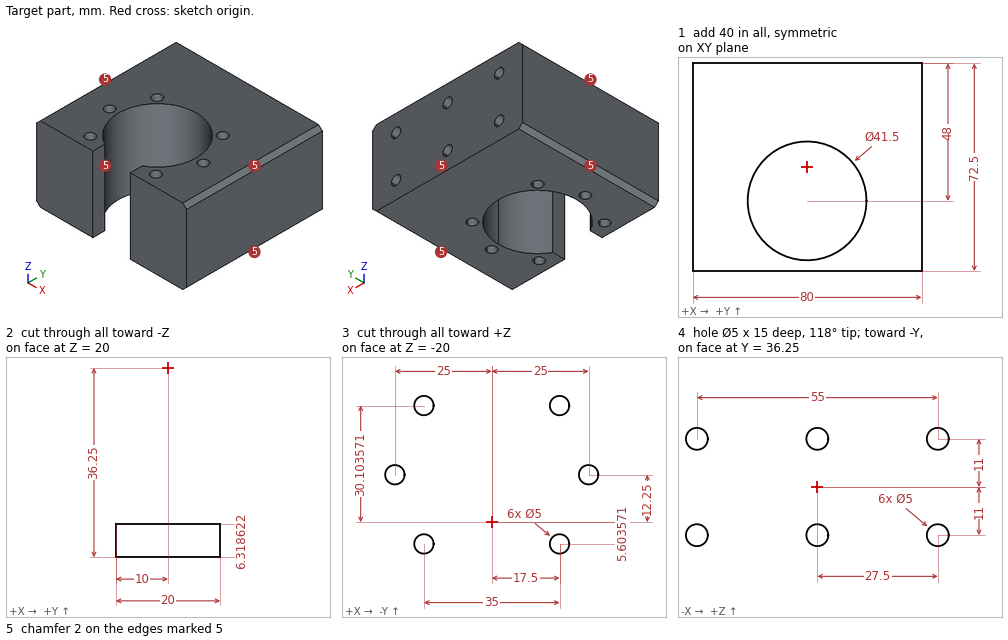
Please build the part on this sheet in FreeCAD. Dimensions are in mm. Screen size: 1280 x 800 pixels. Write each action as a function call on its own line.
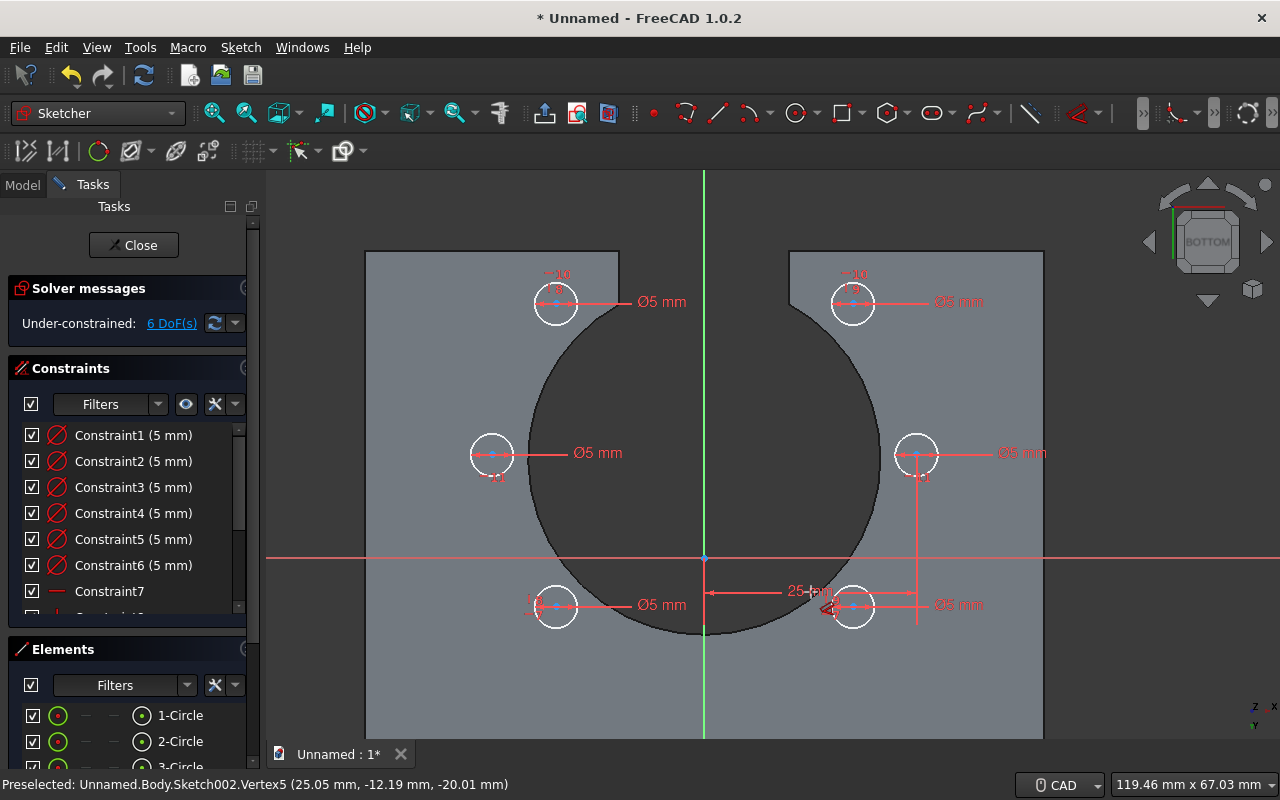
click(492, 455)
click(598, 592)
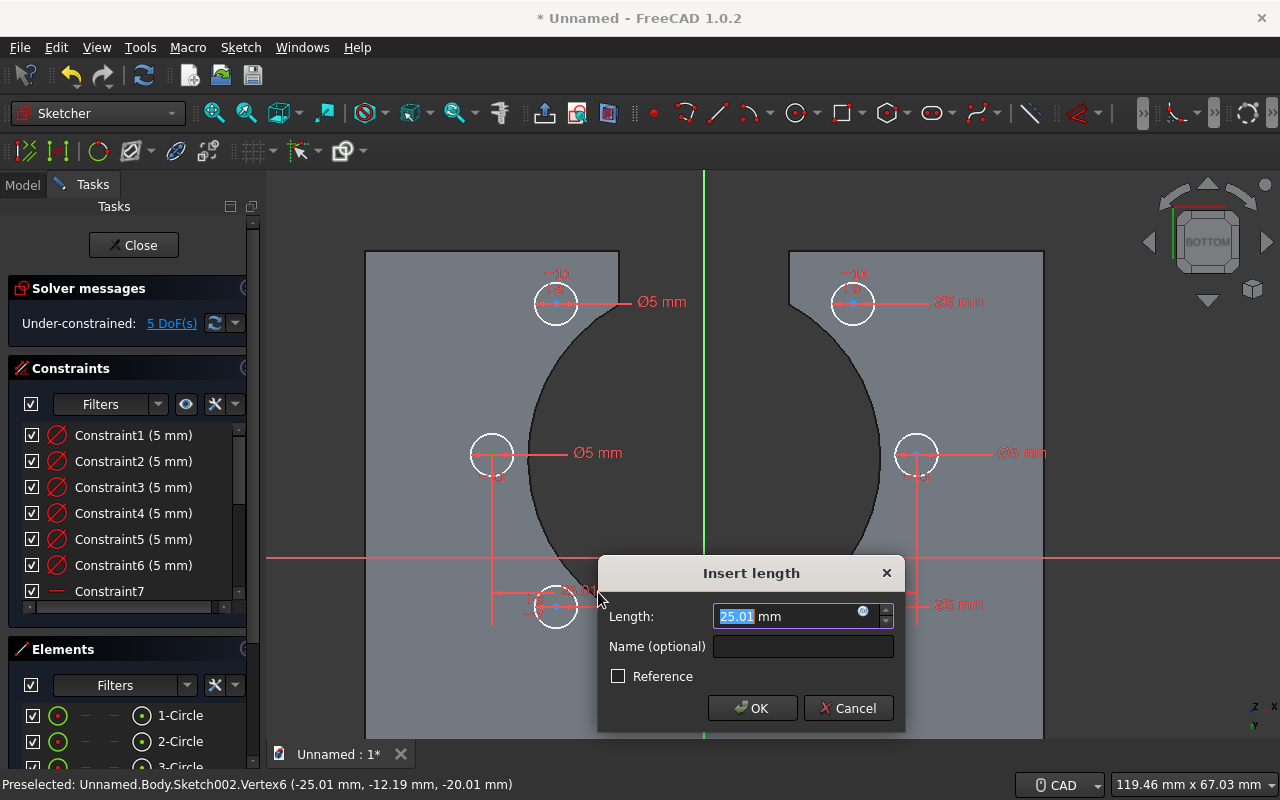
text(25)
key(Return)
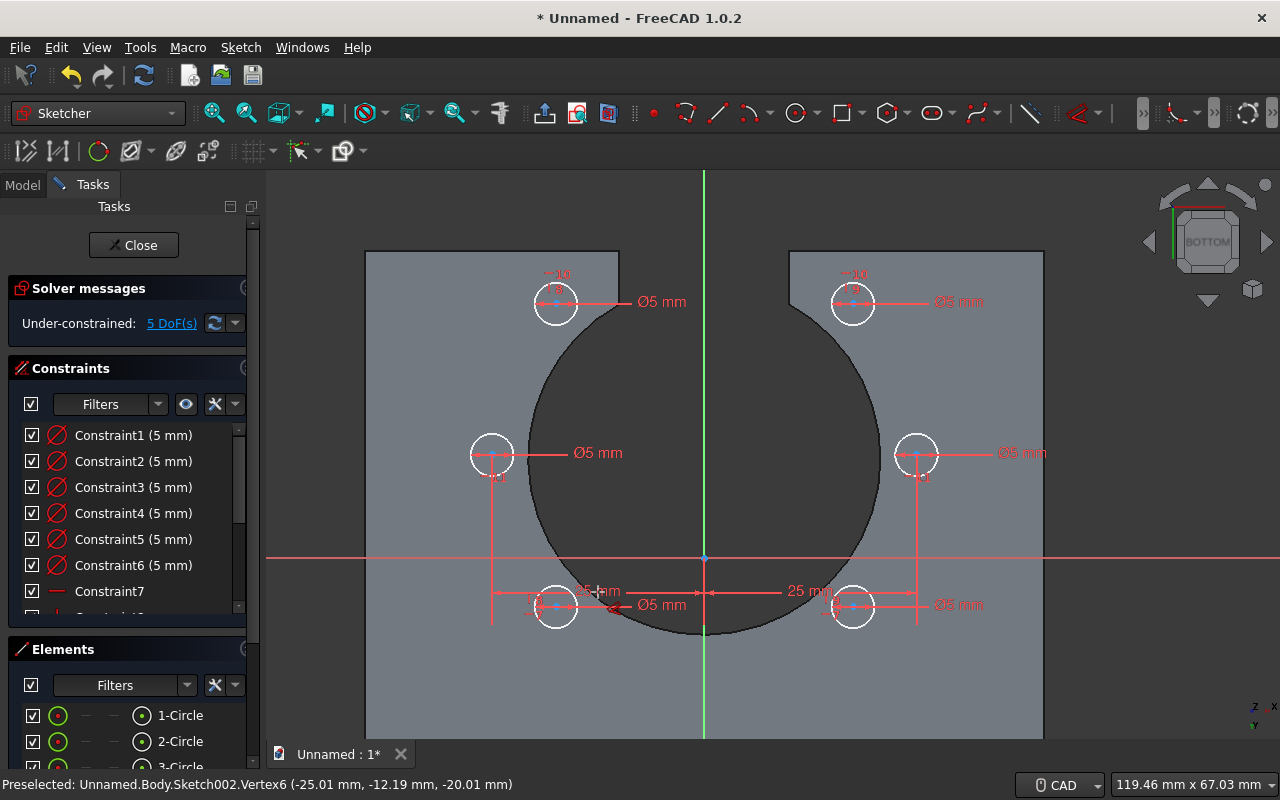
click(853, 607)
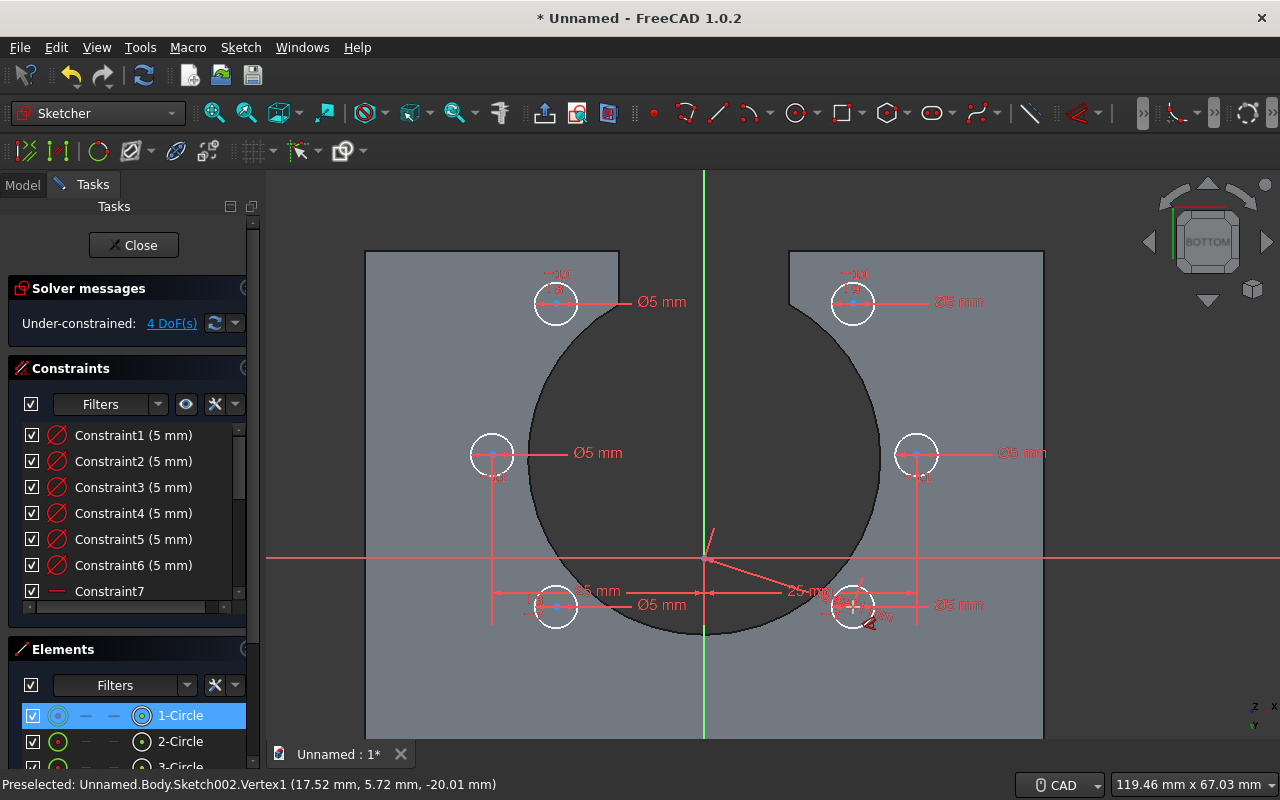
click(556, 607)
click(636, 641)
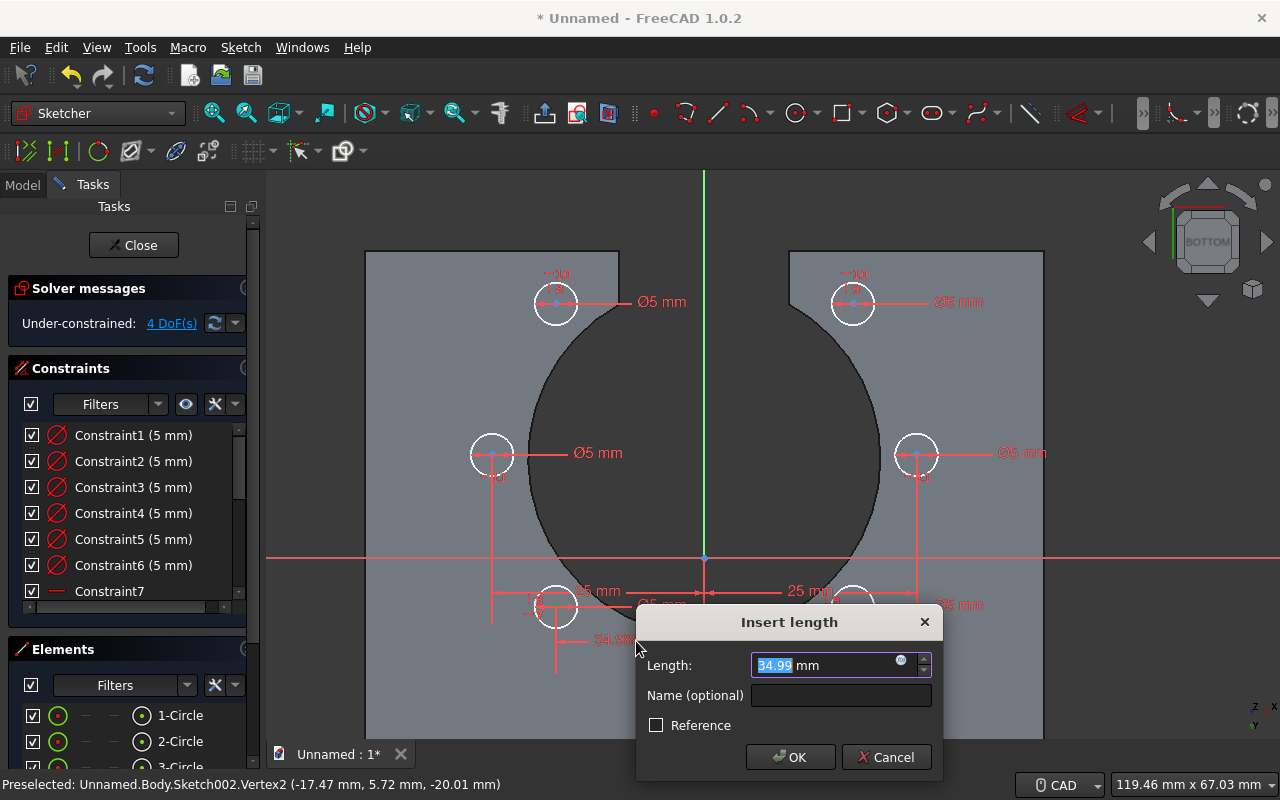
text(35)
key(Return)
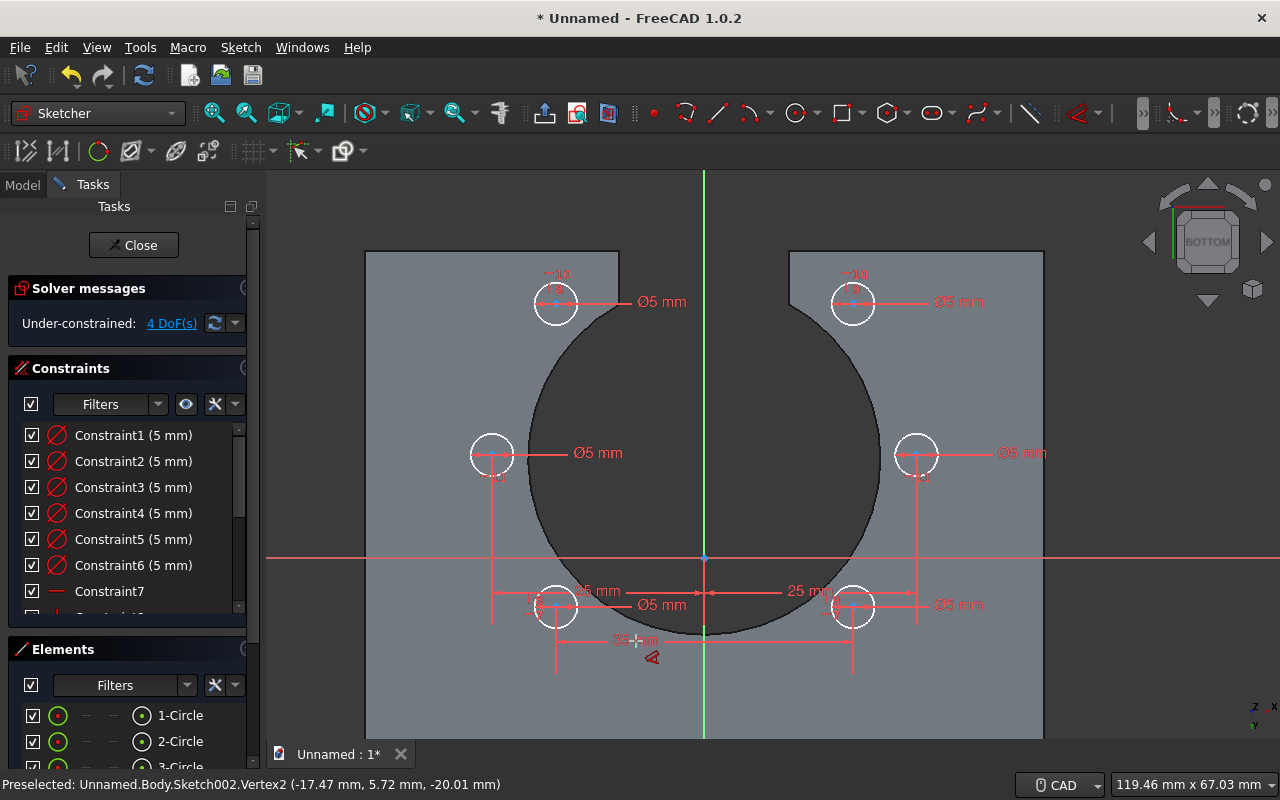
click(853, 607)
click(779, 641)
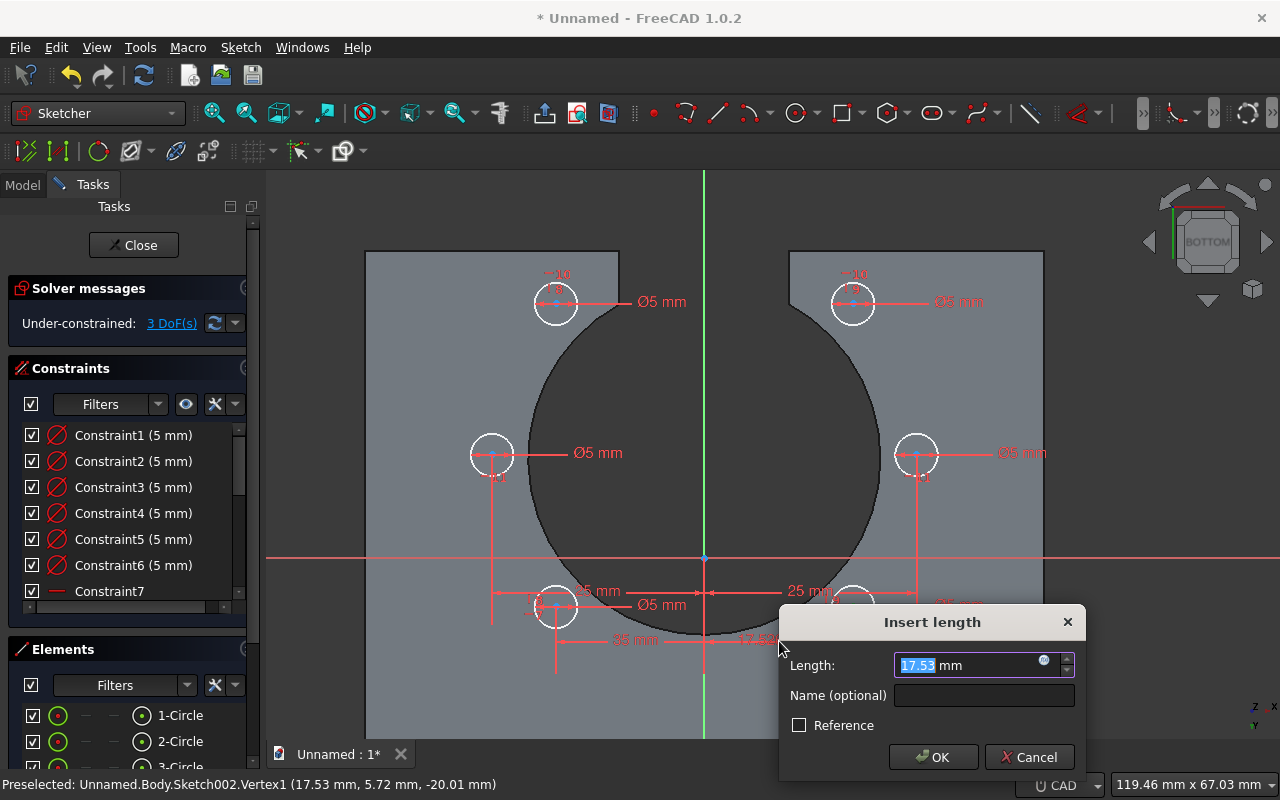
text(17.5)
key(Return)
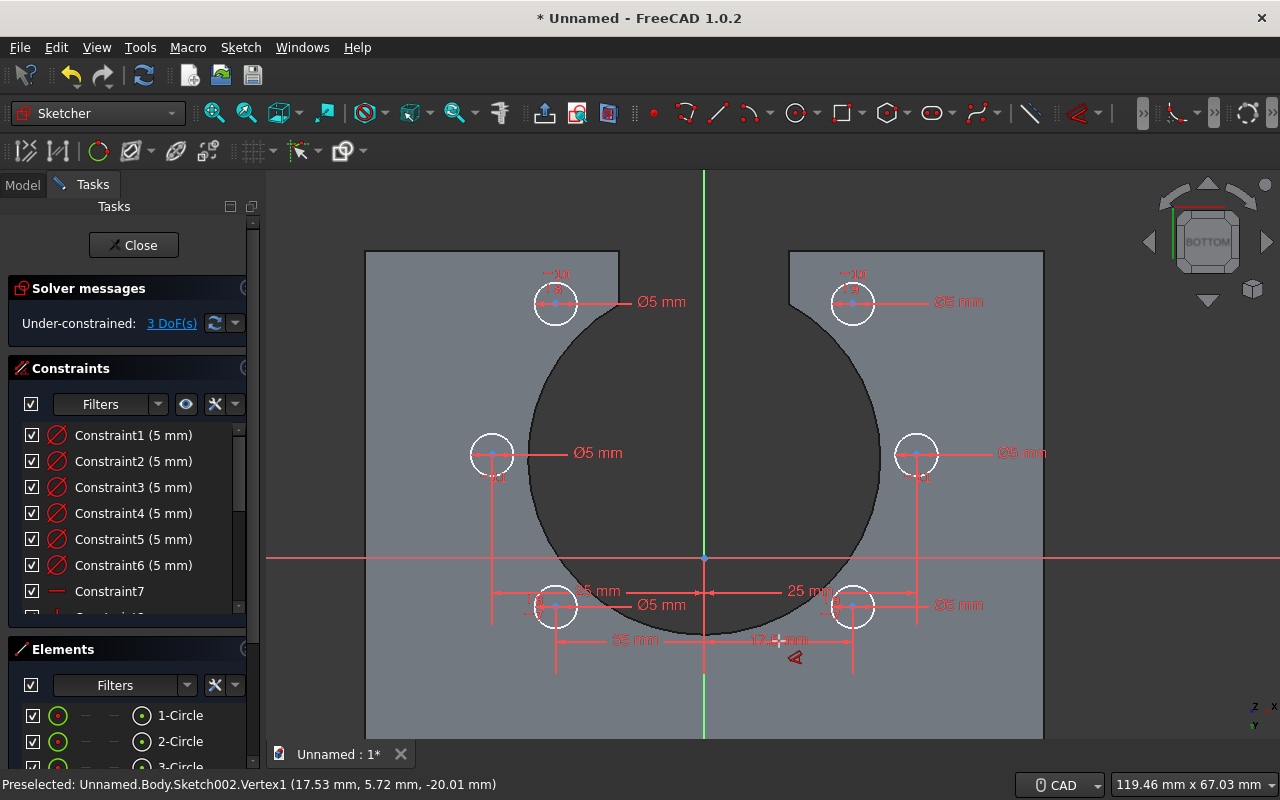
click(917, 455)
click(951, 507)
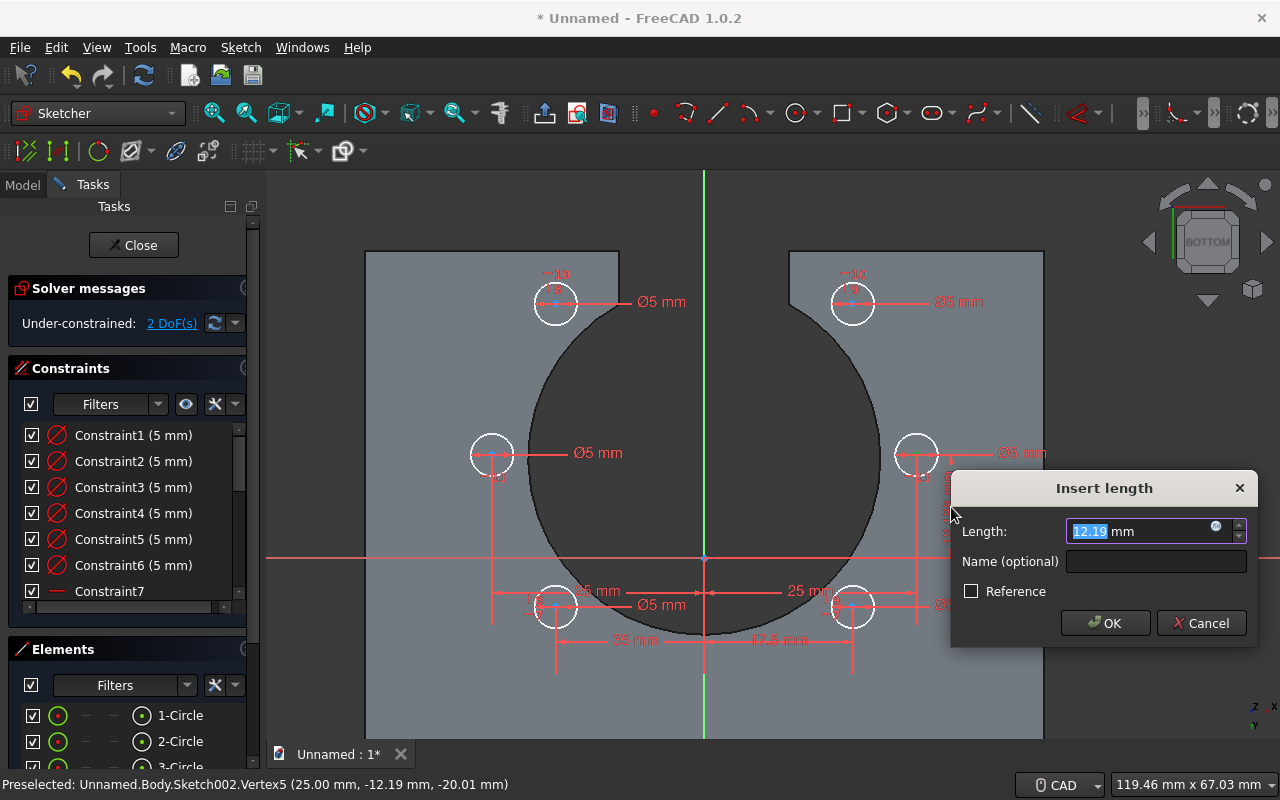
text(12.25)
key(Return)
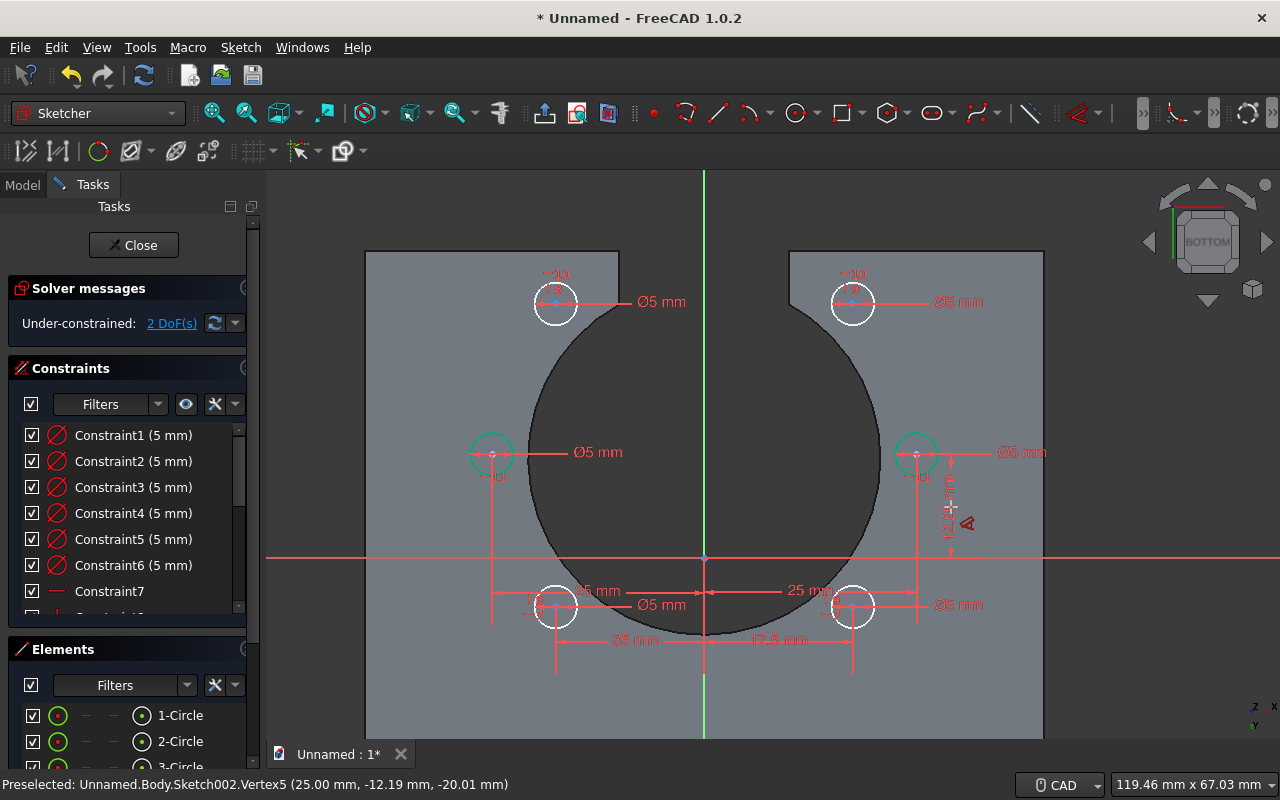
click(853, 607)
click(887, 583)